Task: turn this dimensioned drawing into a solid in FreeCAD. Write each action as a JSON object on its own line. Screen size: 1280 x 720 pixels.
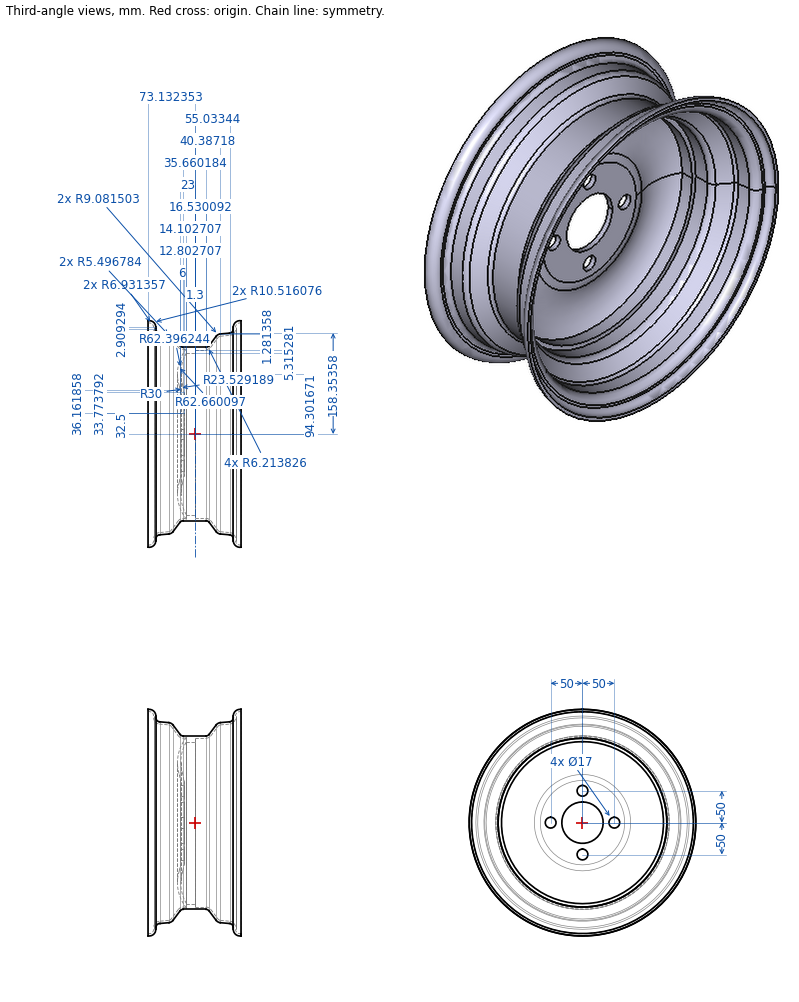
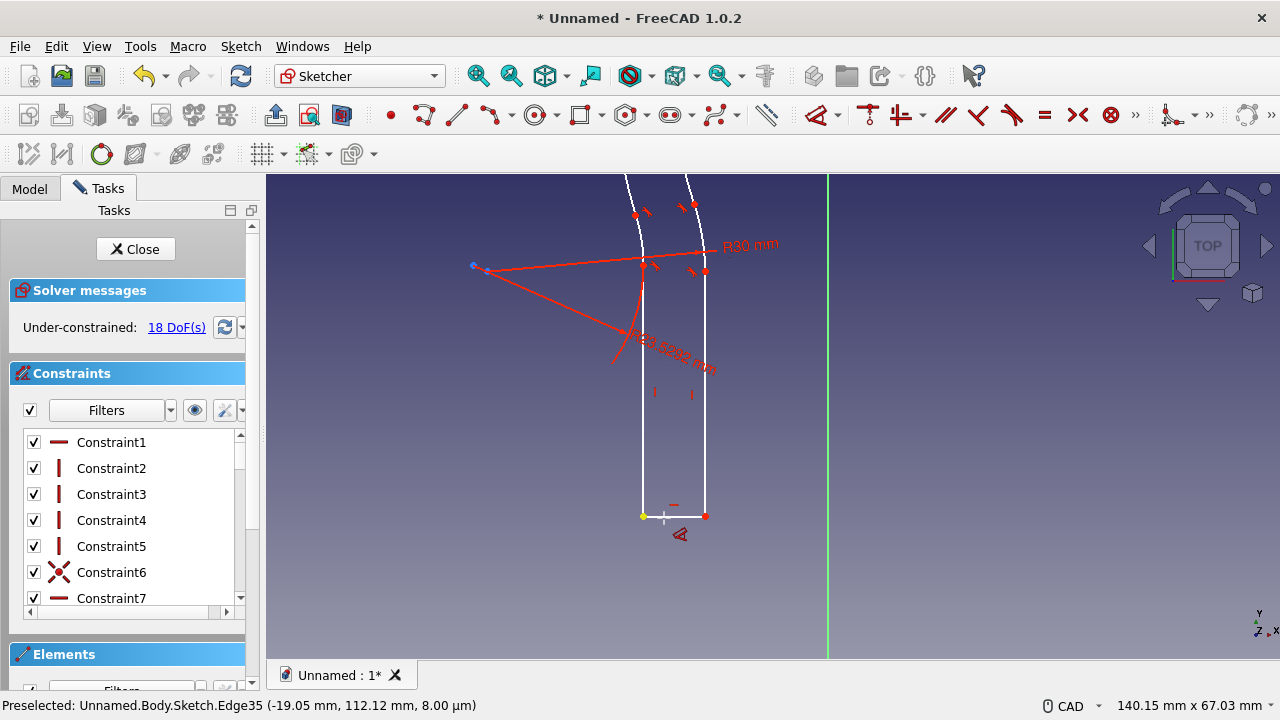
{"action": "left_click", "coordinate": [662, 517]}
{"action": "left_click", "coordinate": [674, 551]}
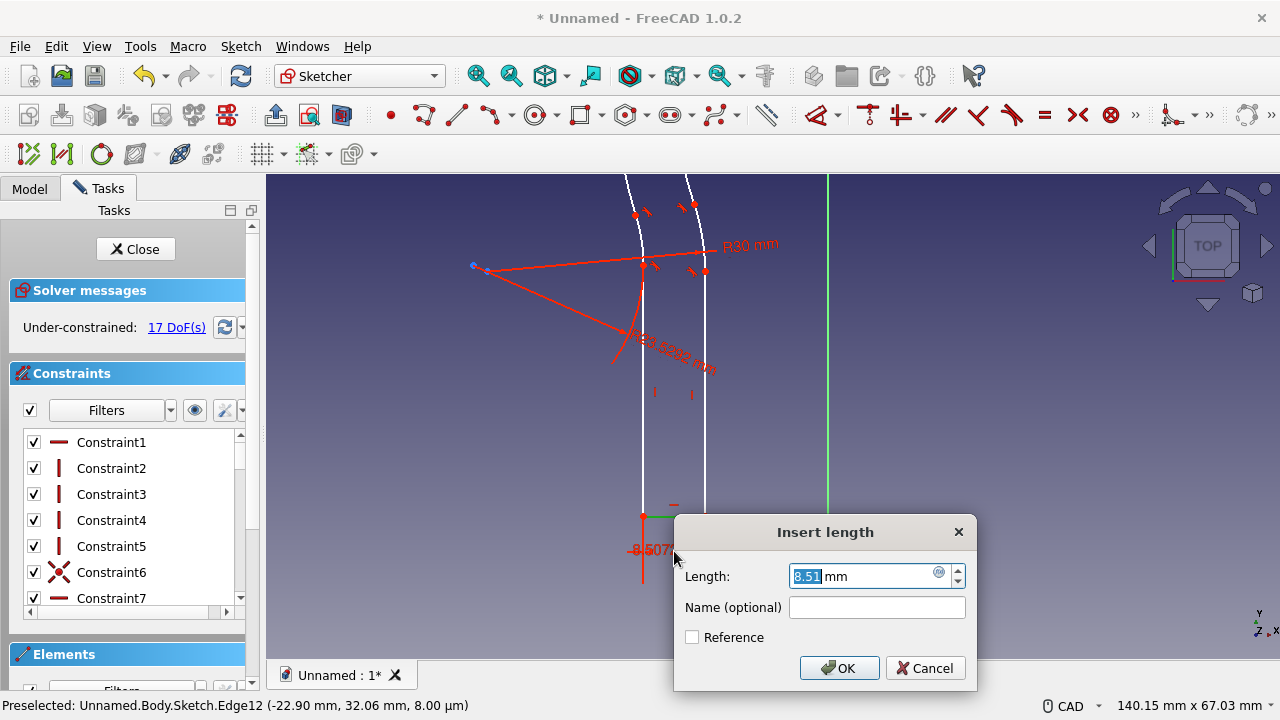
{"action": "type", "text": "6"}
{"action": "key", "text": "Return"}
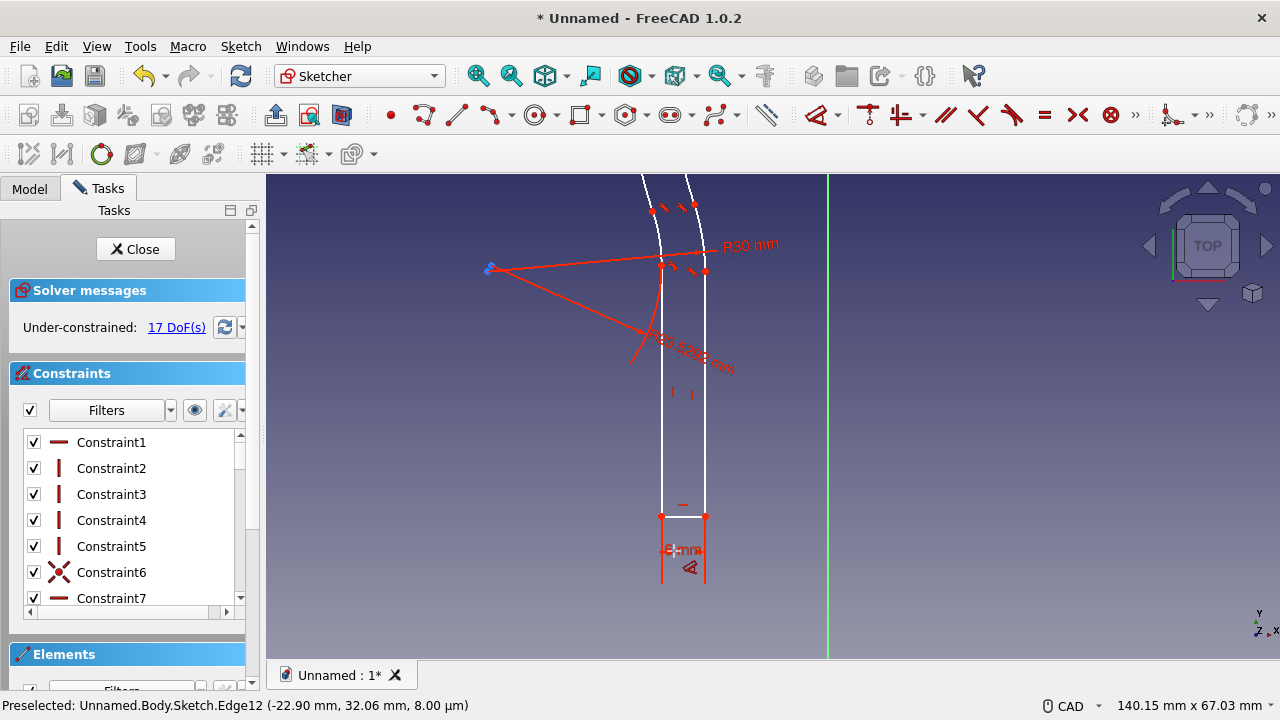
{"action": "scroll", "coordinate": [664, 518], "scroll_direction": "down", "scroll_amount": 7}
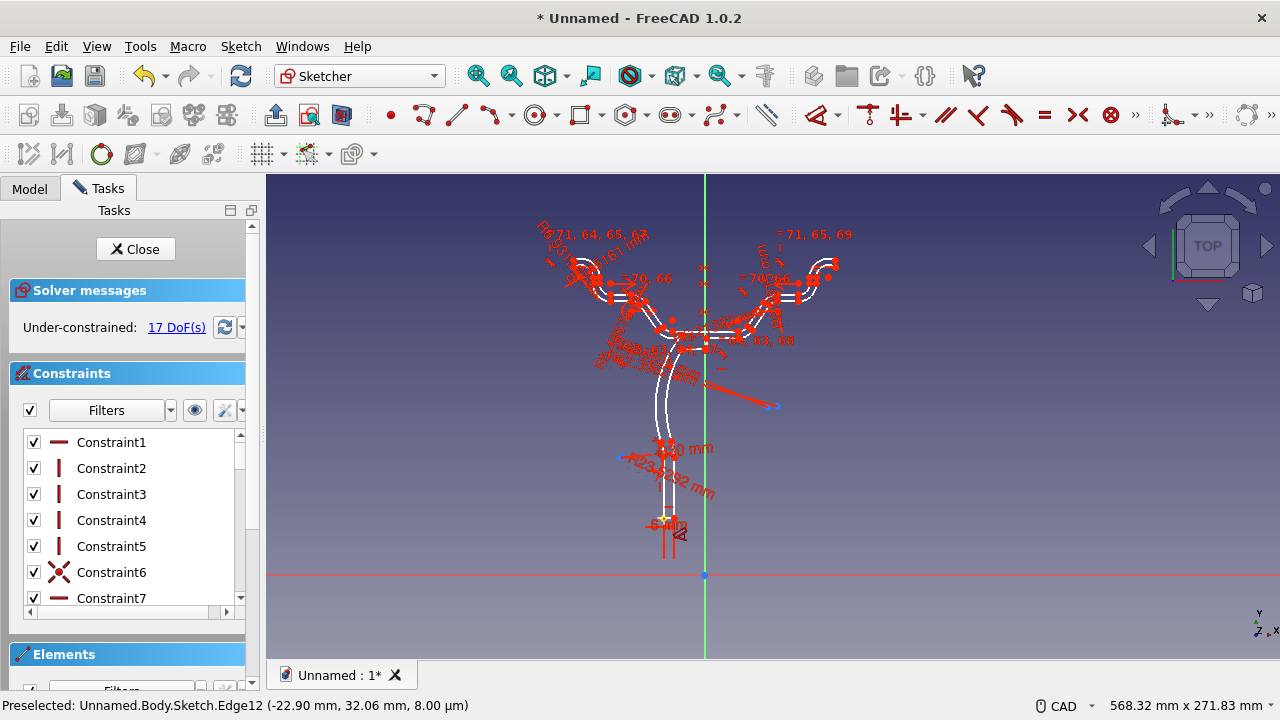
{"action": "left_click", "coordinate": [664, 456]}
{"action": "left_click", "coordinate": [684, 609]}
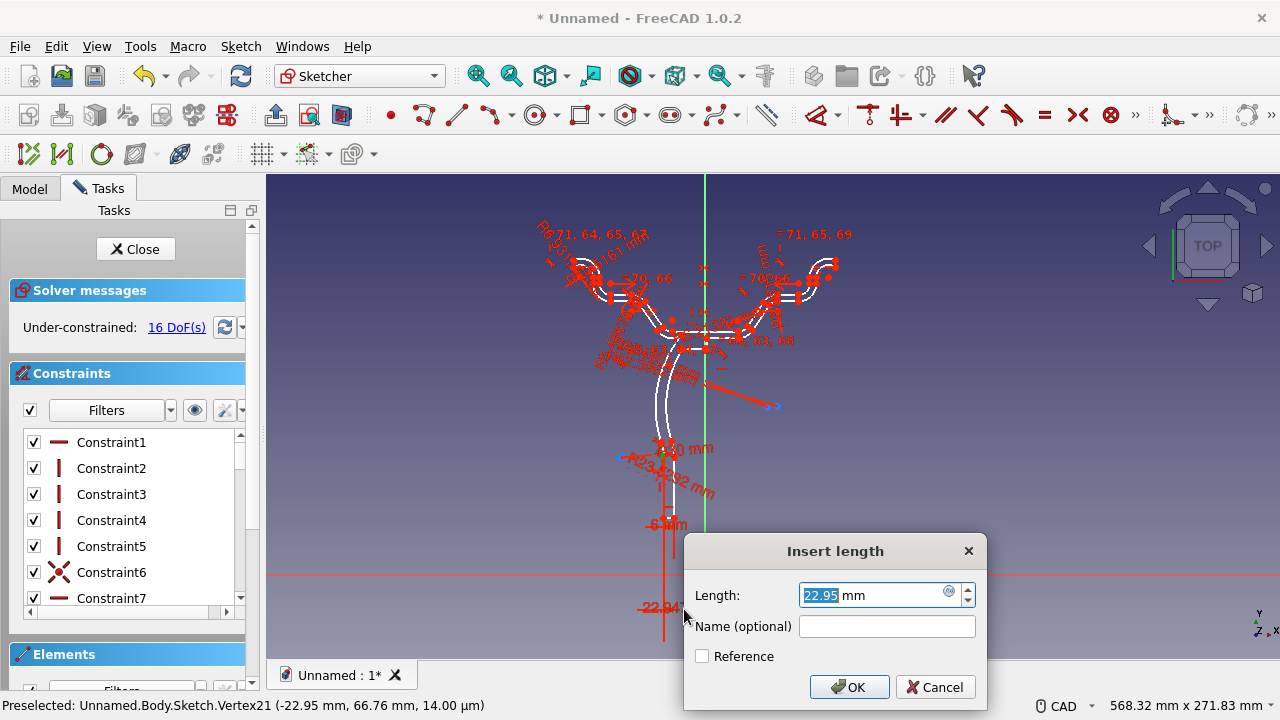
{"action": "type", "text": "23"}
{"action": "key", "text": "Return"}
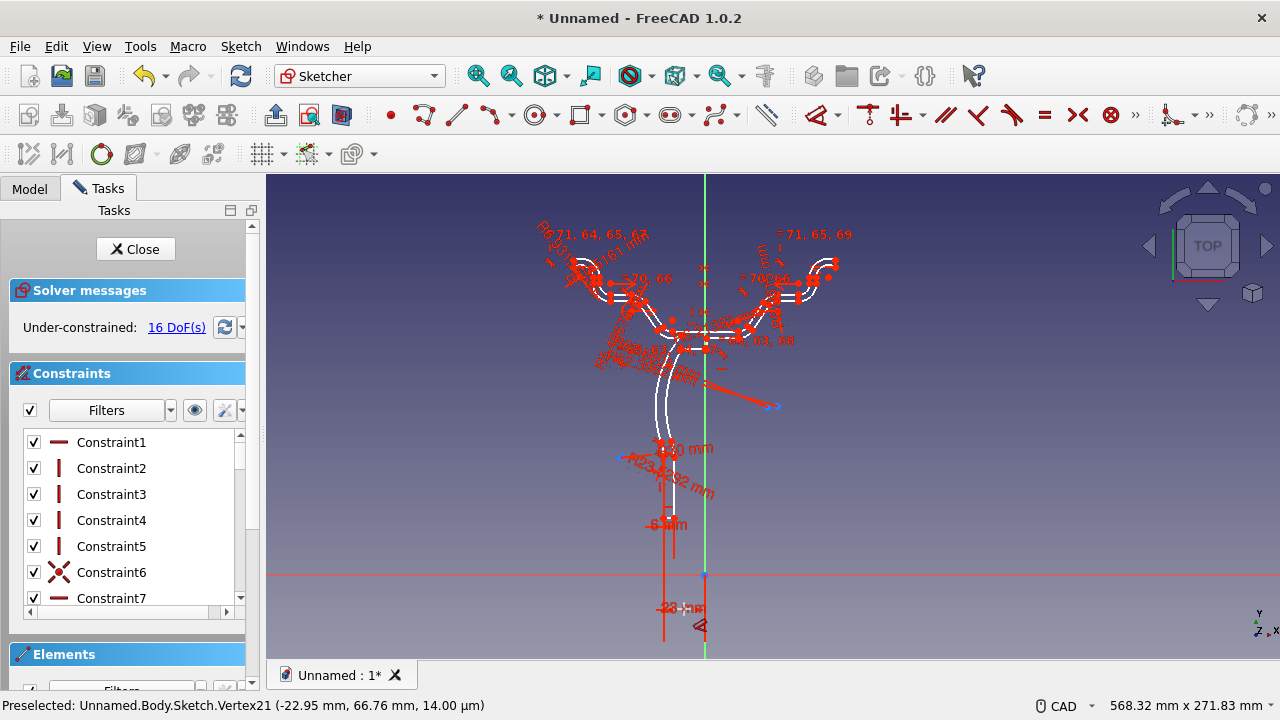
{"action": "scroll", "coordinate": [707, 349], "scroll_direction": "up", "scroll_amount": 15}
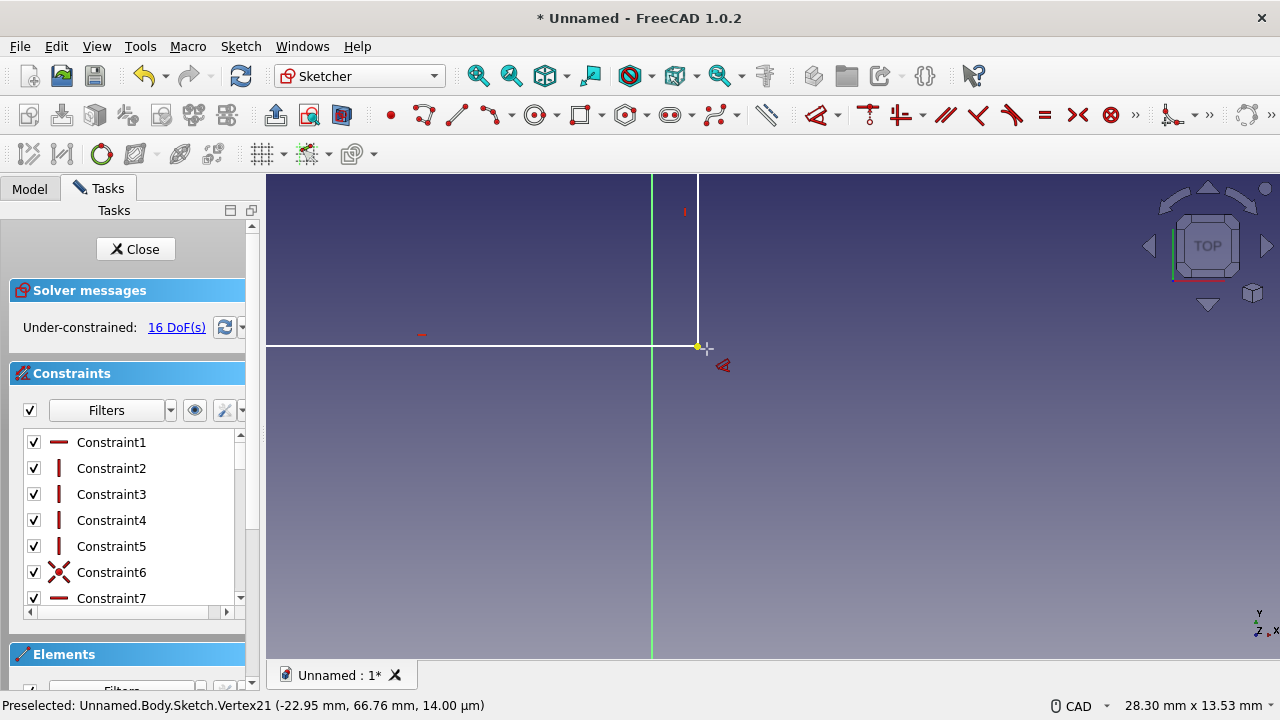
{"action": "left_click", "coordinate": [698, 346]}
{"action": "left_click", "coordinate": [675, 312]}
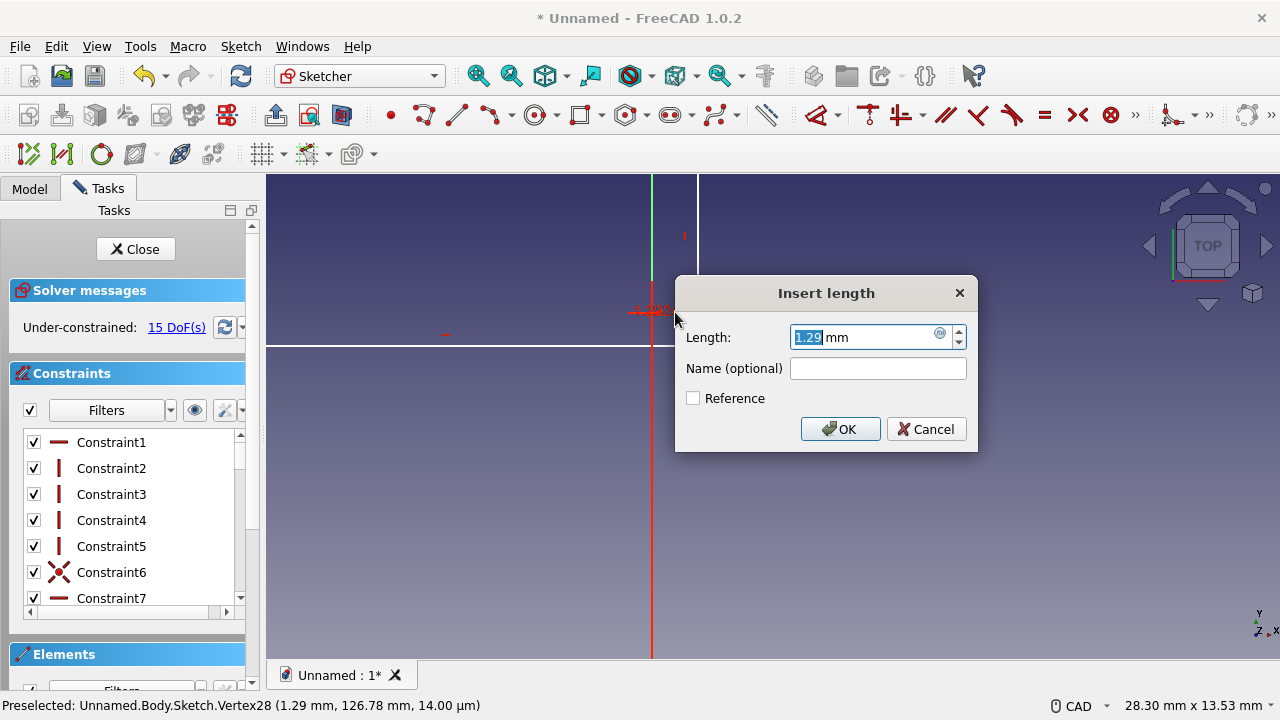
{"action": "type", "text": "1.3"}
{"action": "key", "text": "Return"}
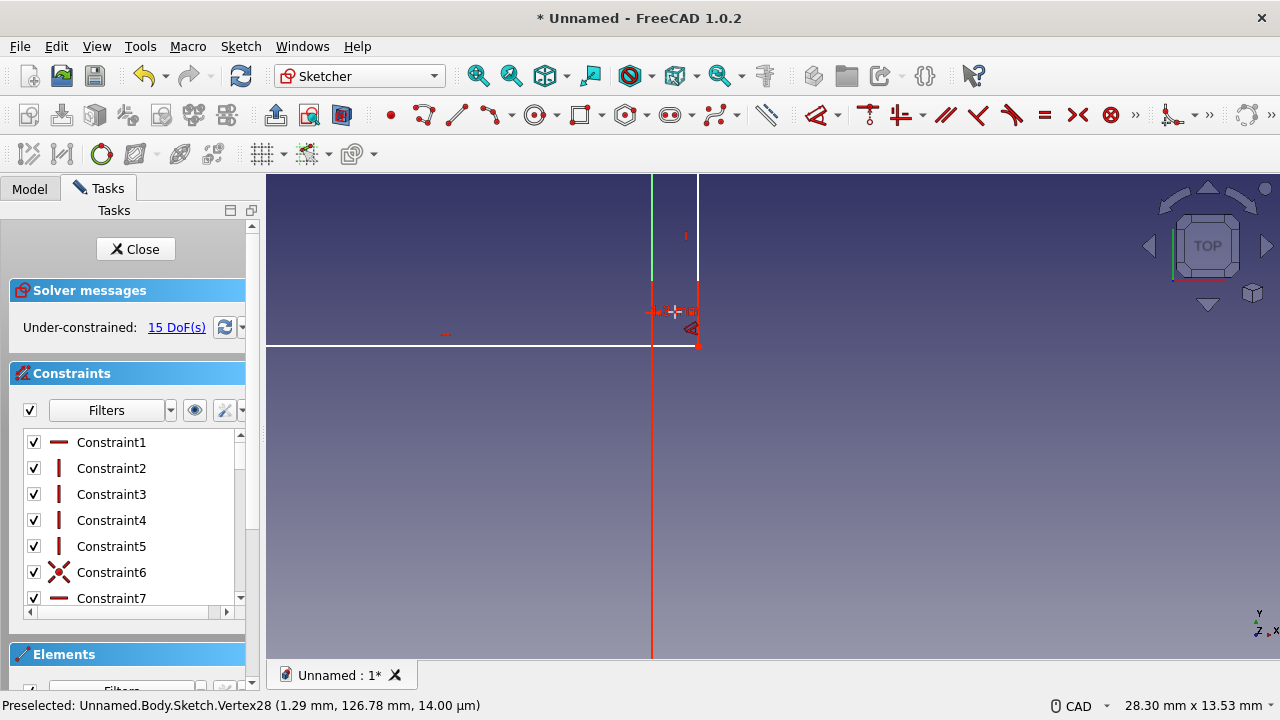
{"action": "scroll", "coordinate": [707, 349], "scroll_direction": "down", "scroll_amount": 15}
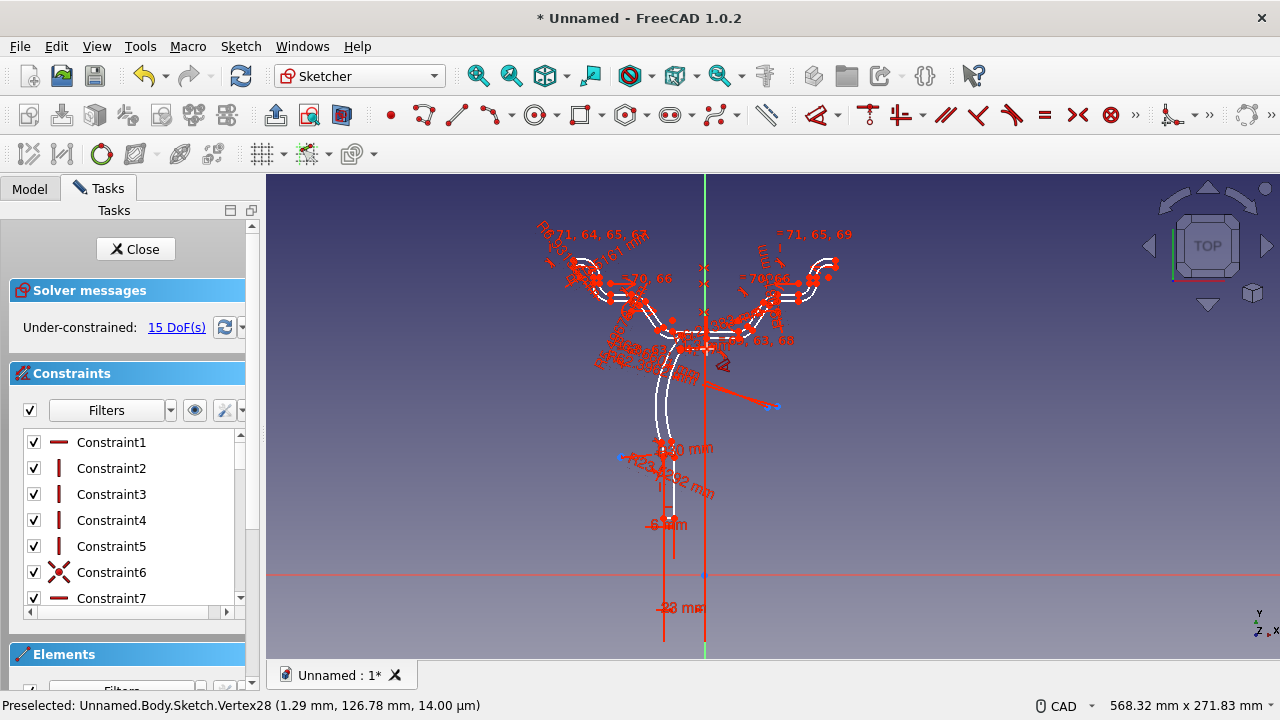
{"action": "left_click", "coordinate": [664, 518]}
{"action": "left_click", "coordinate": [630, 547]}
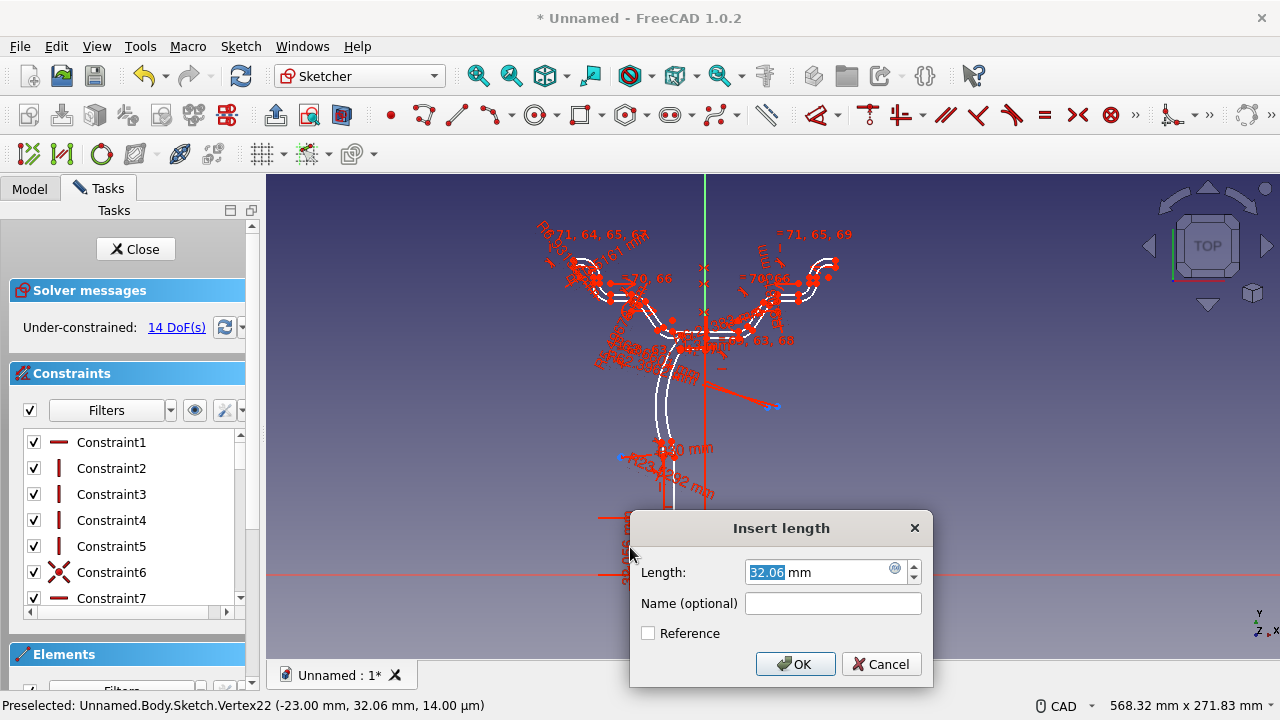
{"action": "type", "text": "32.5"}
{"action": "key", "text": "Return"}